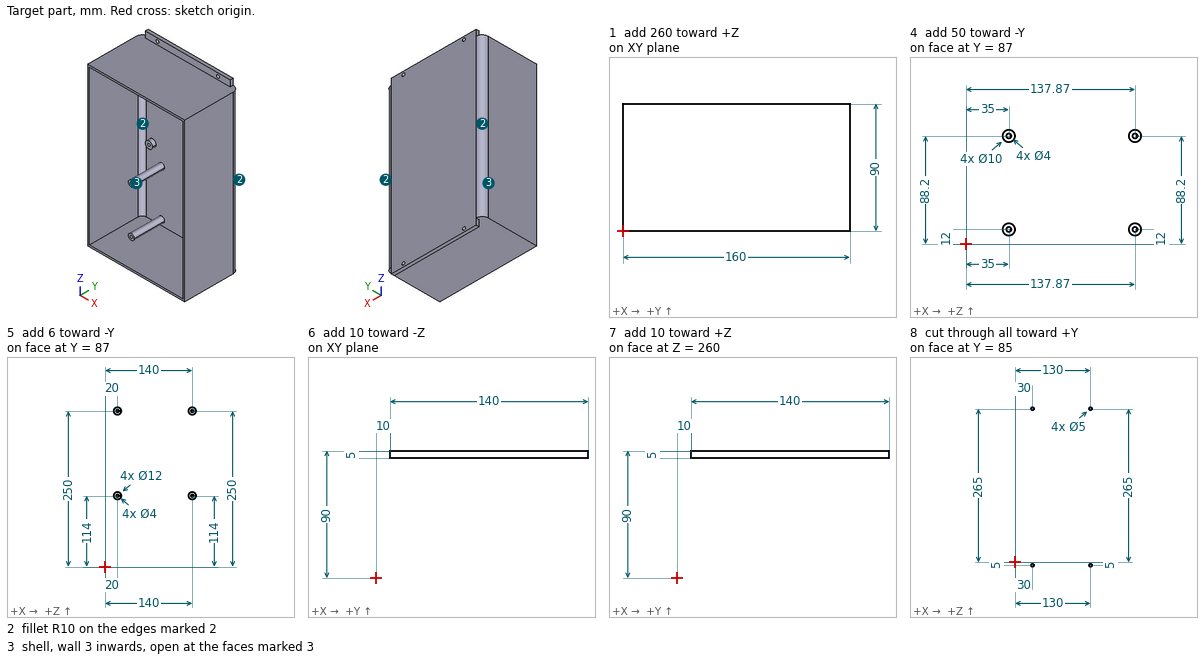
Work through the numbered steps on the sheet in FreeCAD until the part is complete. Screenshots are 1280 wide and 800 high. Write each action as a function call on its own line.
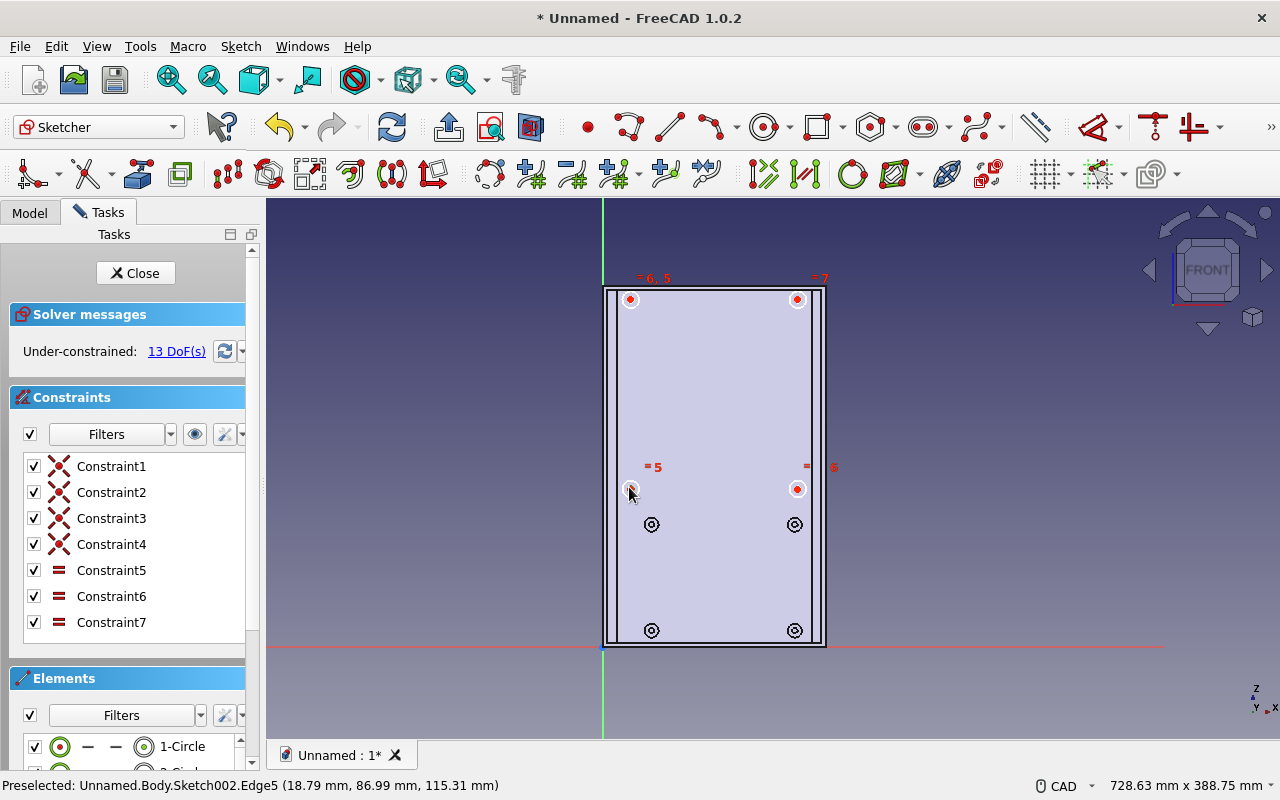
scroll(633, 298, up, 8)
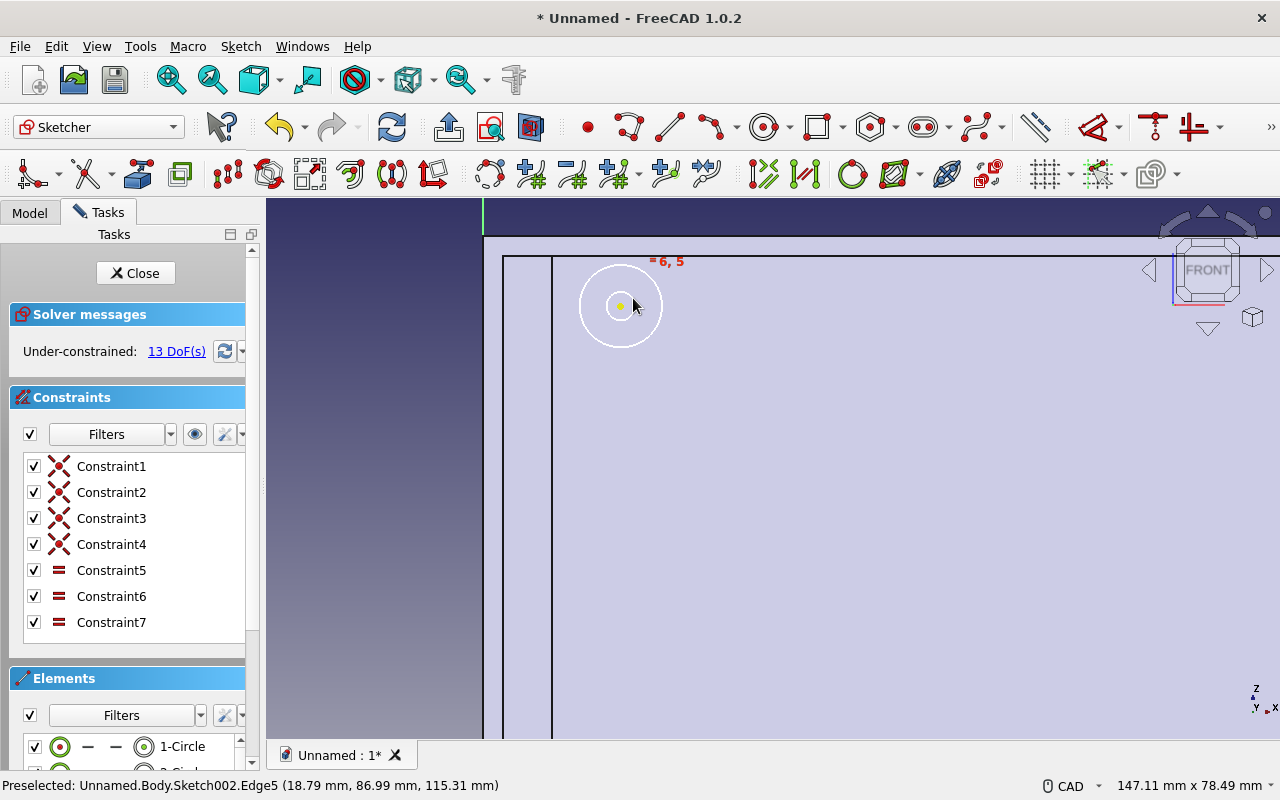
click(631, 296)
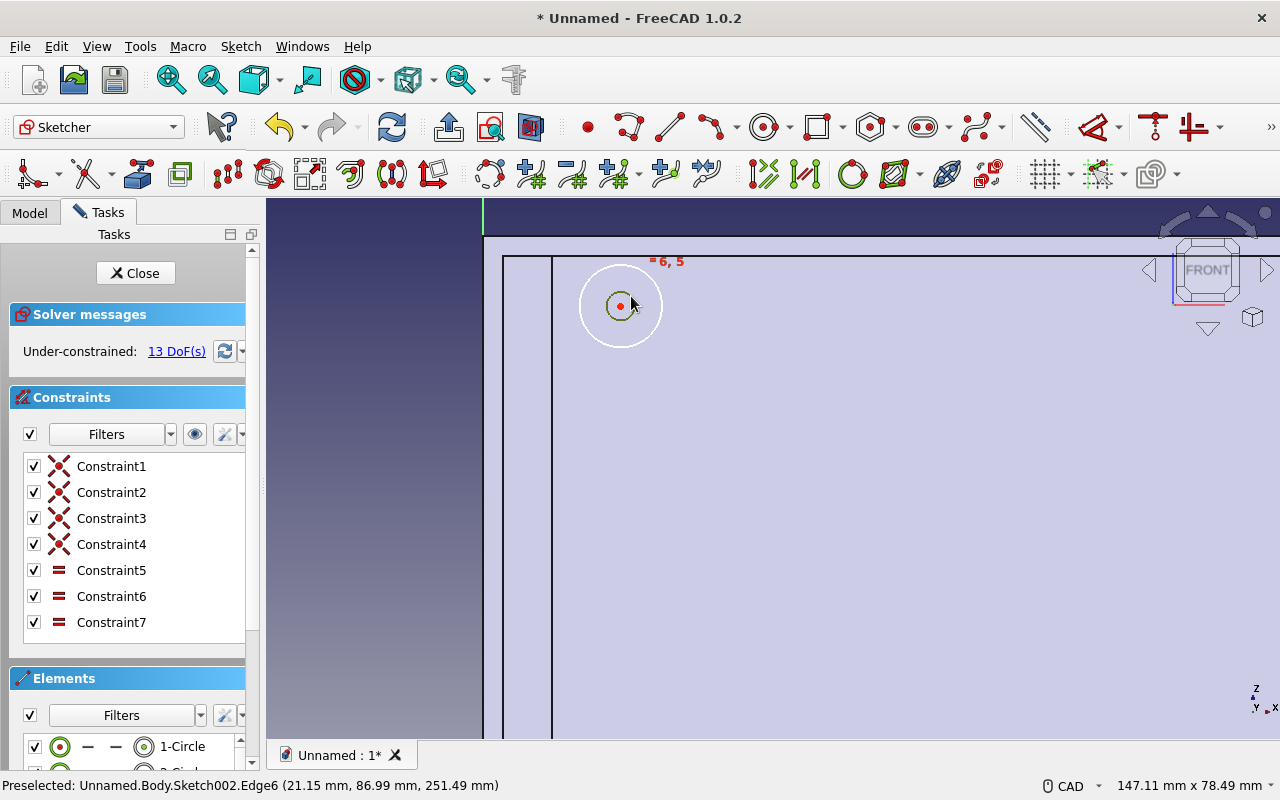
scroll(633, 297, down, 8)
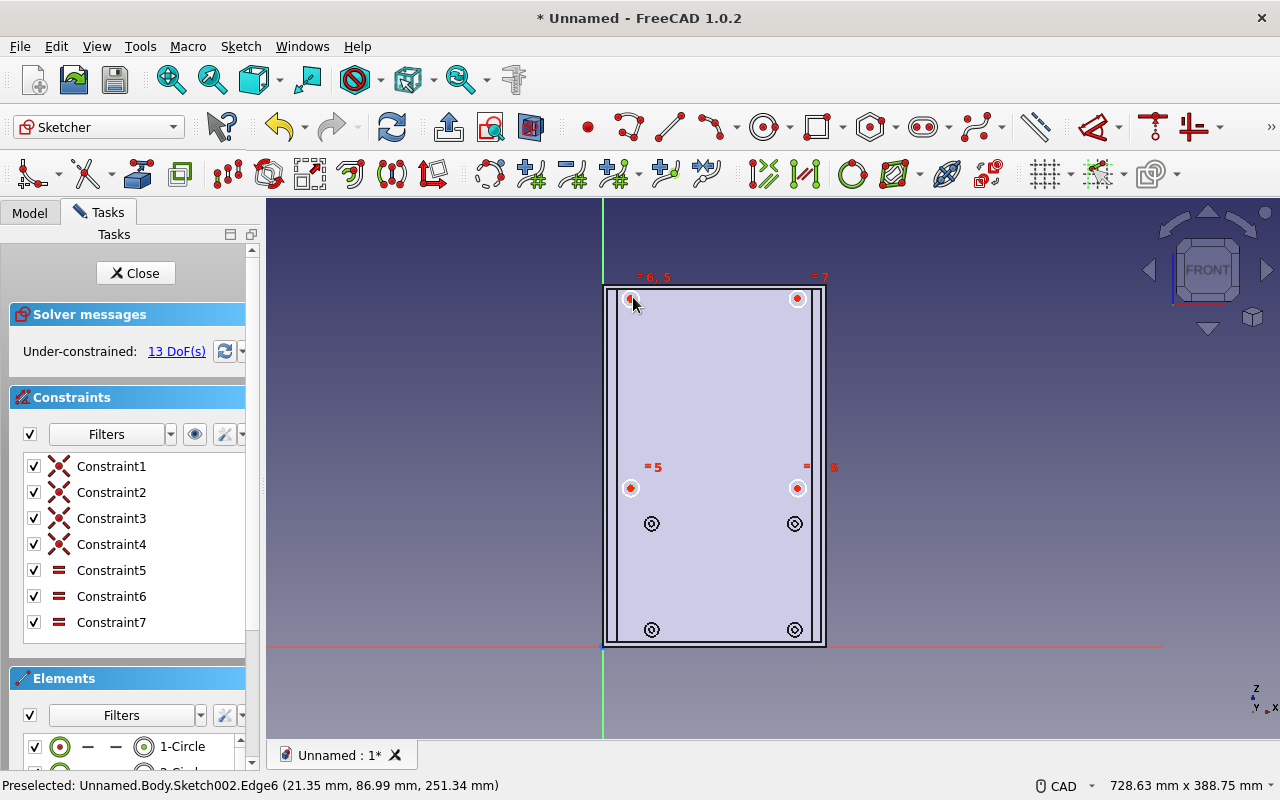
scroll(800, 486, up, 9)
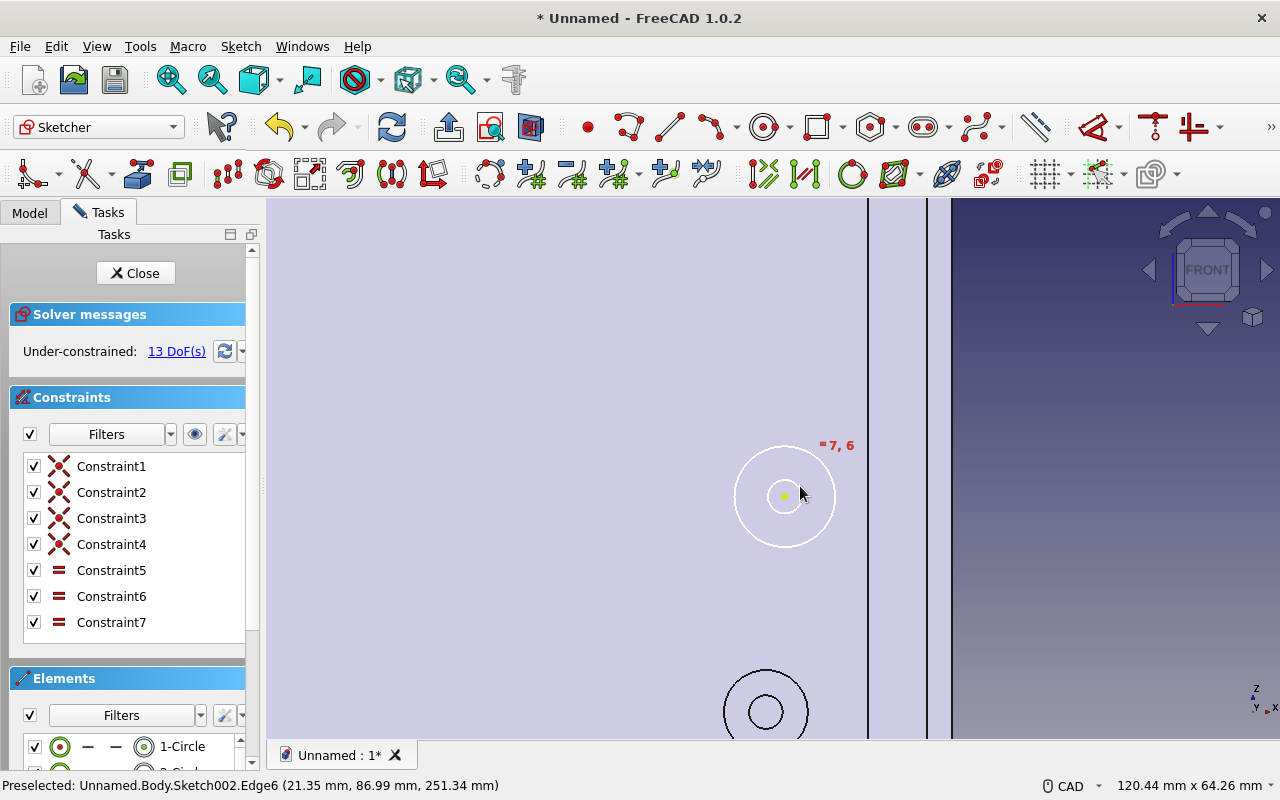
click(797, 485)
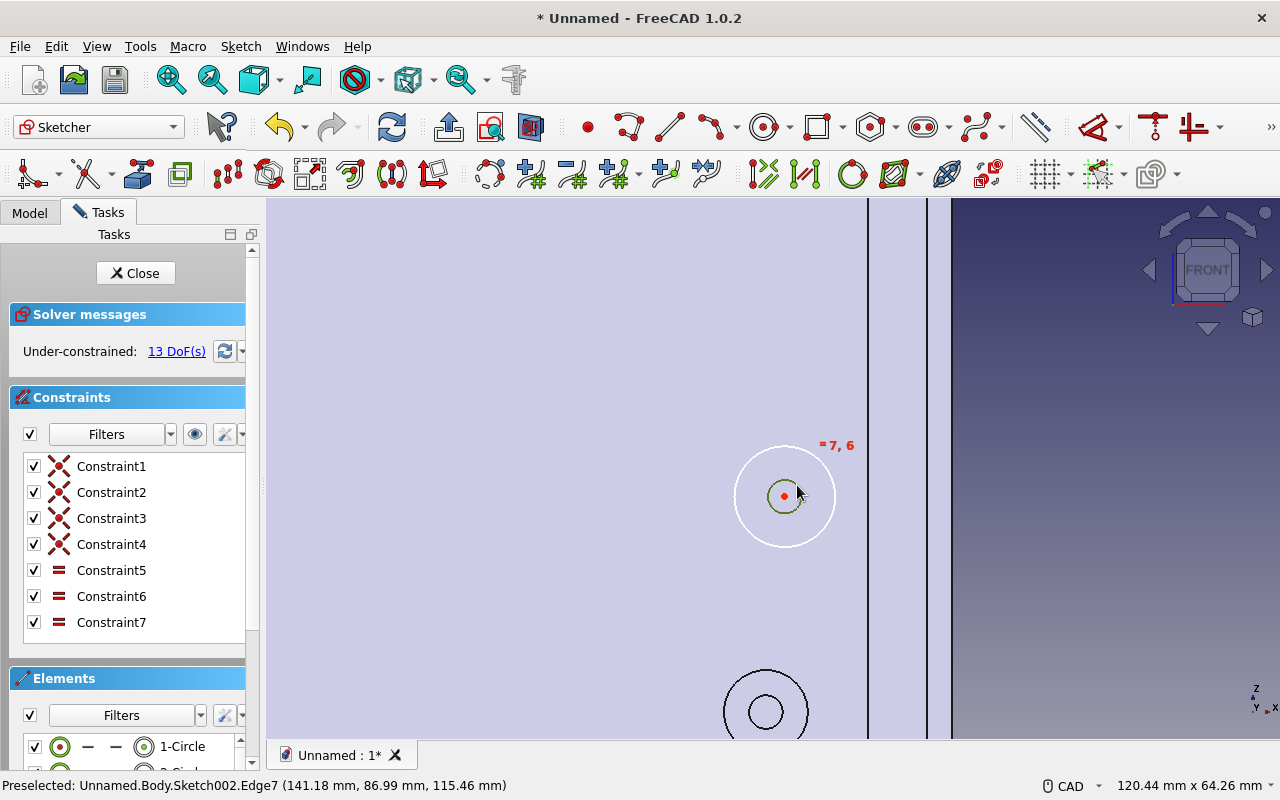
scroll(800, 487, down, 9)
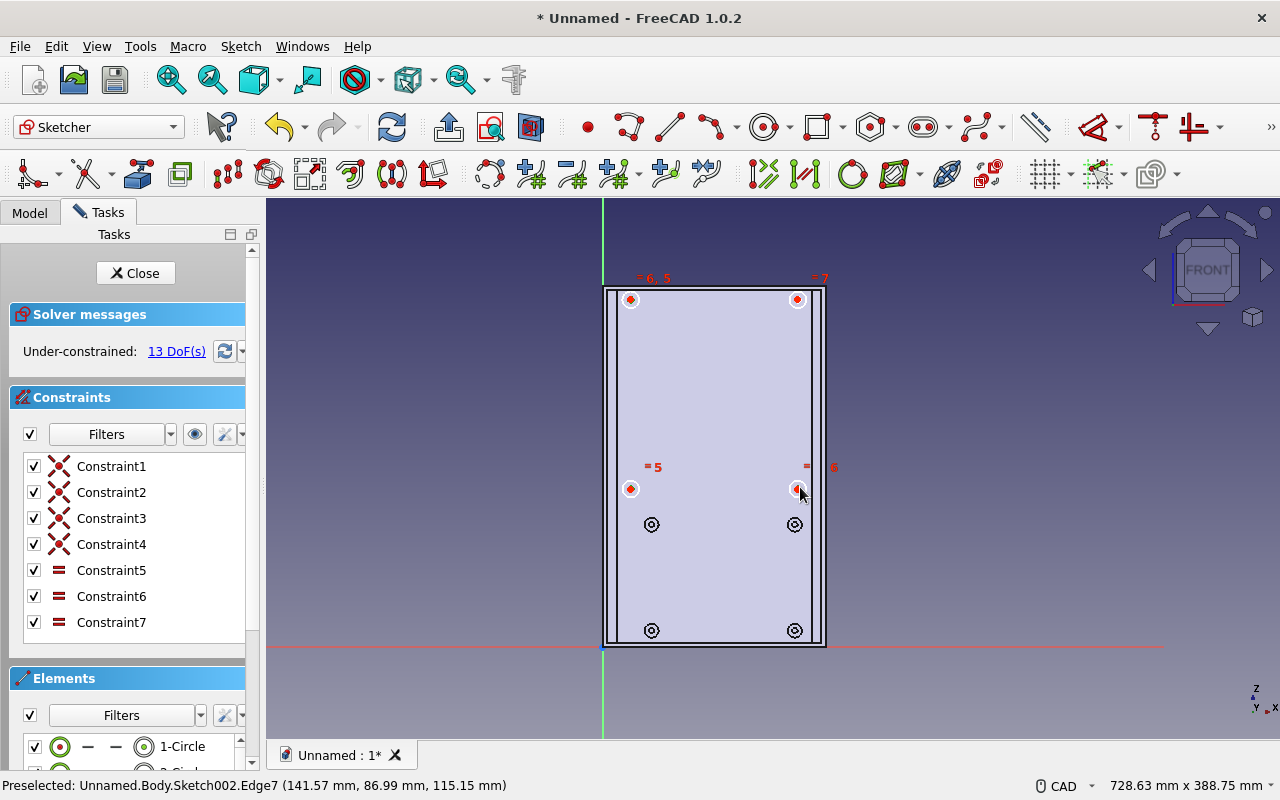
scroll(800, 298, up, 8)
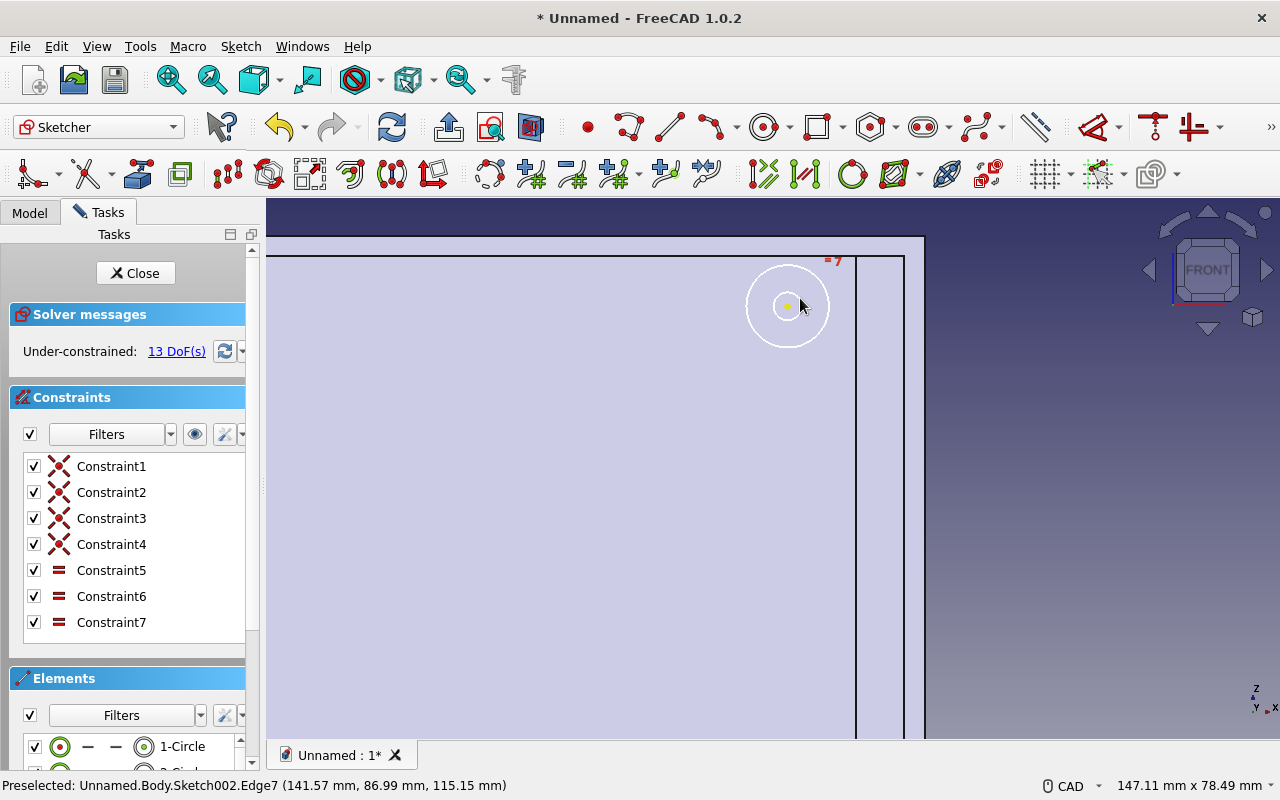
click(798, 296)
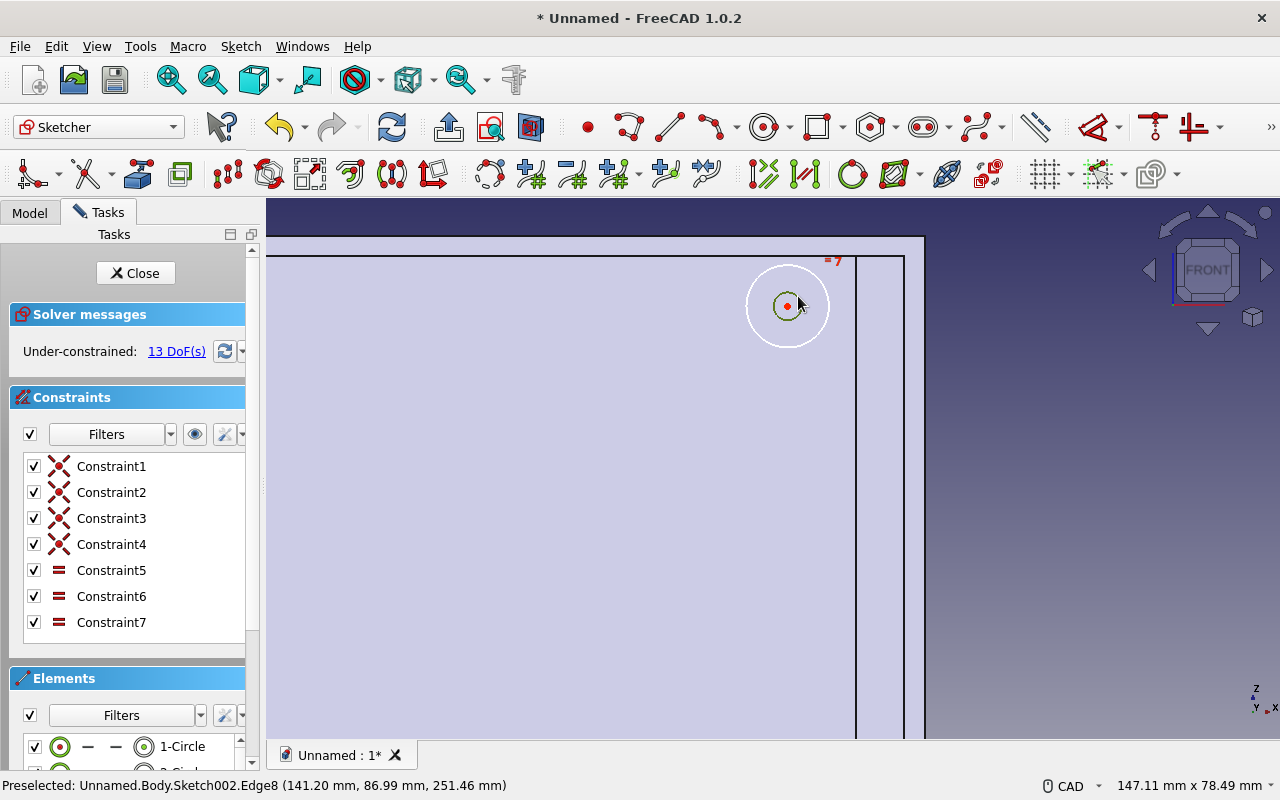
key(e)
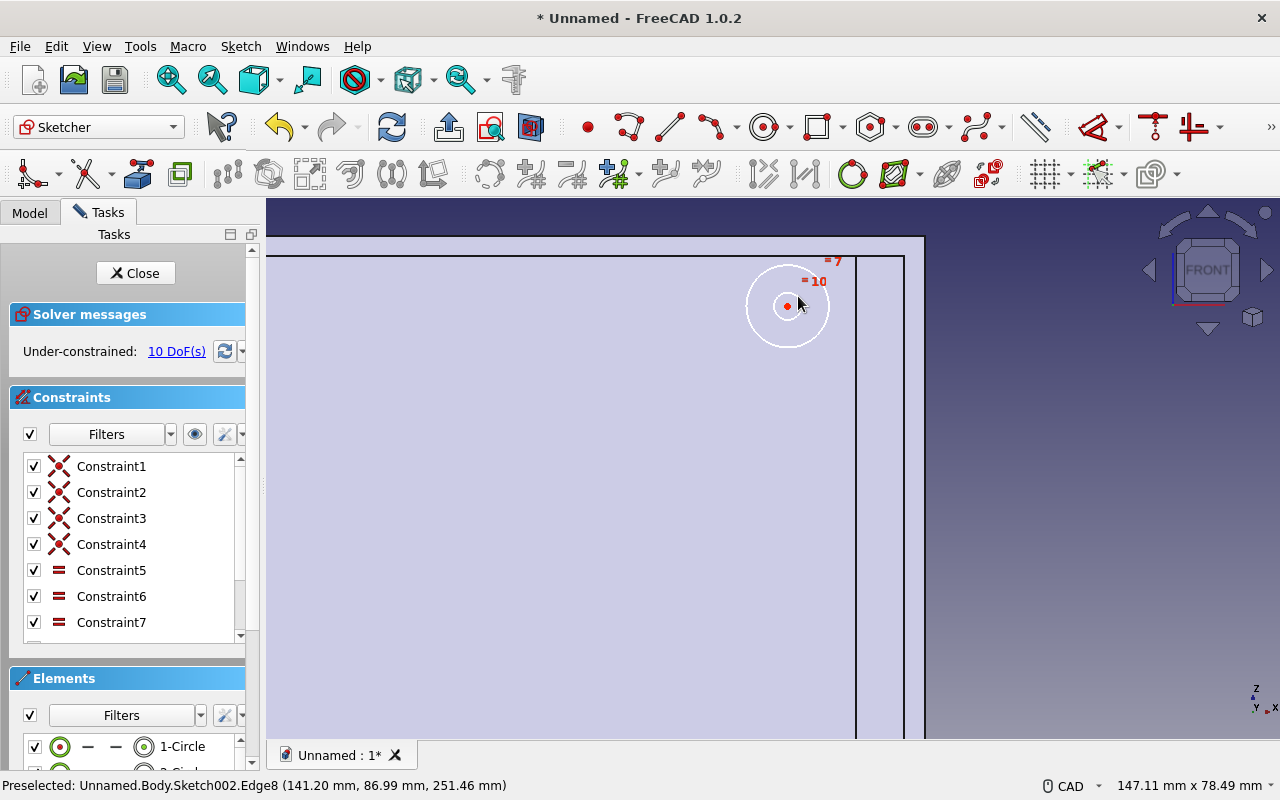
click(1092, 128)